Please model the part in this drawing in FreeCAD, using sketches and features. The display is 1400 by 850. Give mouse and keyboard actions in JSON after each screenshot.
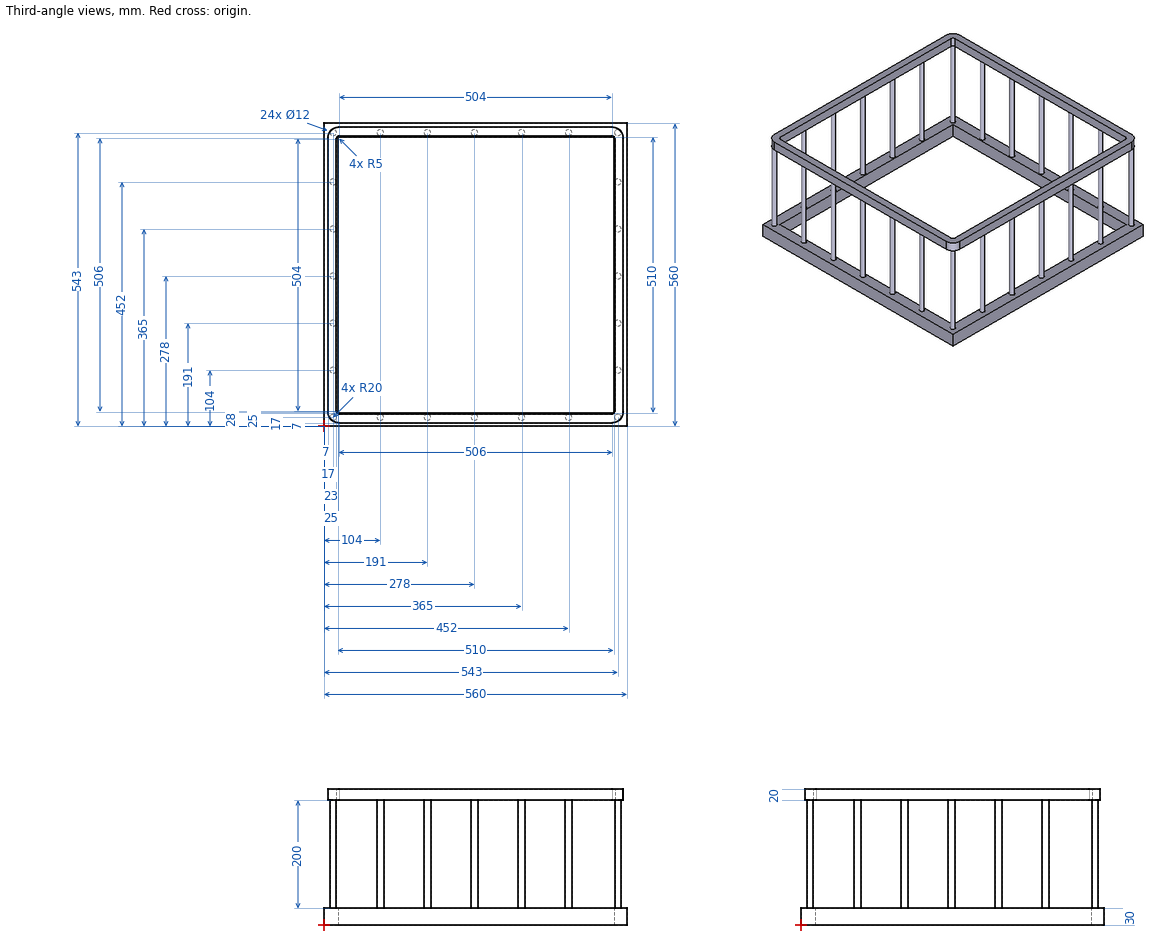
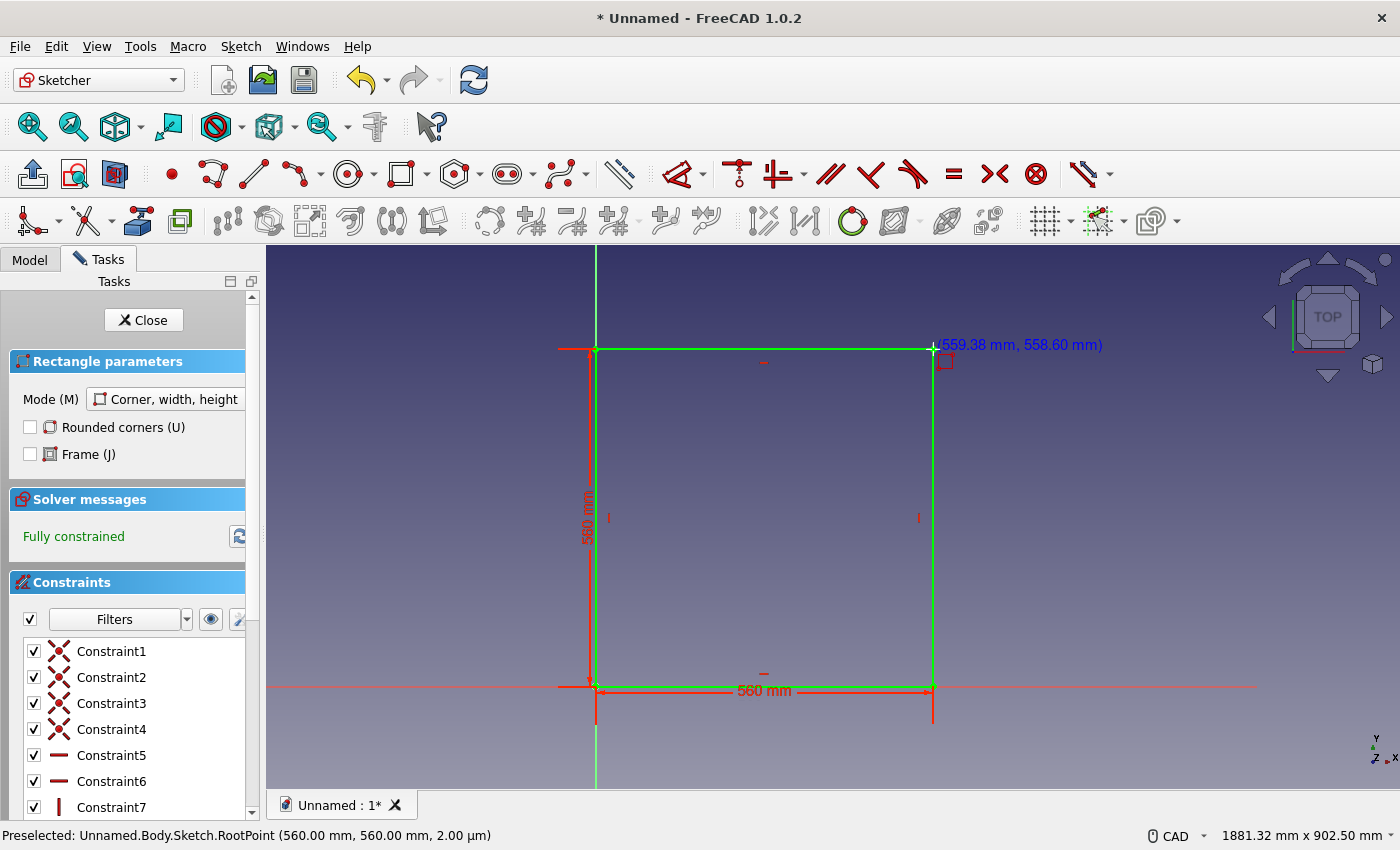
{"action": "left_click", "coordinate": [611, 364]}
{"action": "mouse_move", "coordinate": [918, 672]}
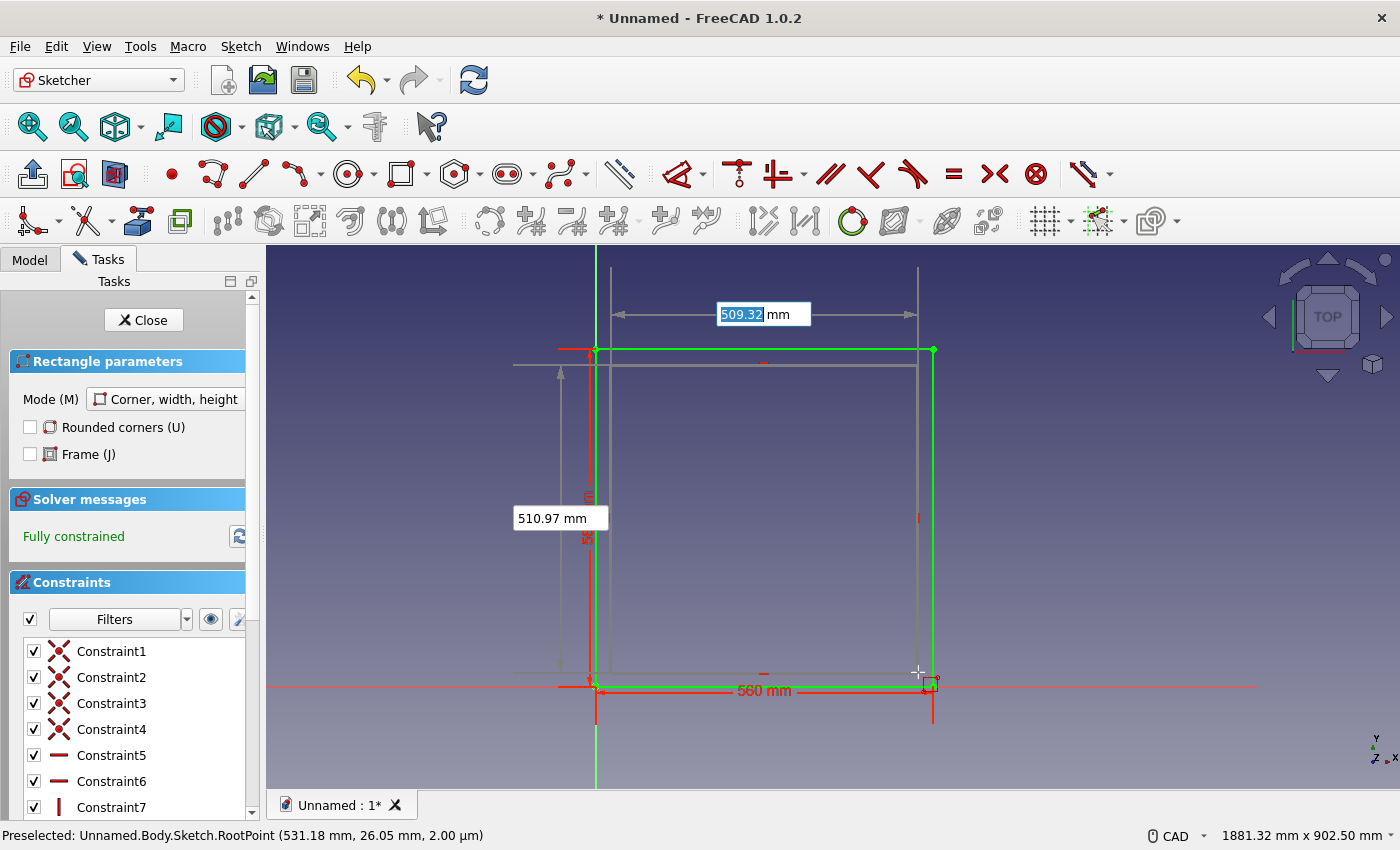
{"action": "type", "text": "510"}
{"action": "key", "text": "Tab"}
{"action": "type", "text": "510"}
{"action": "key", "text": "Return"}
{"action": "key", "text": "Escape"}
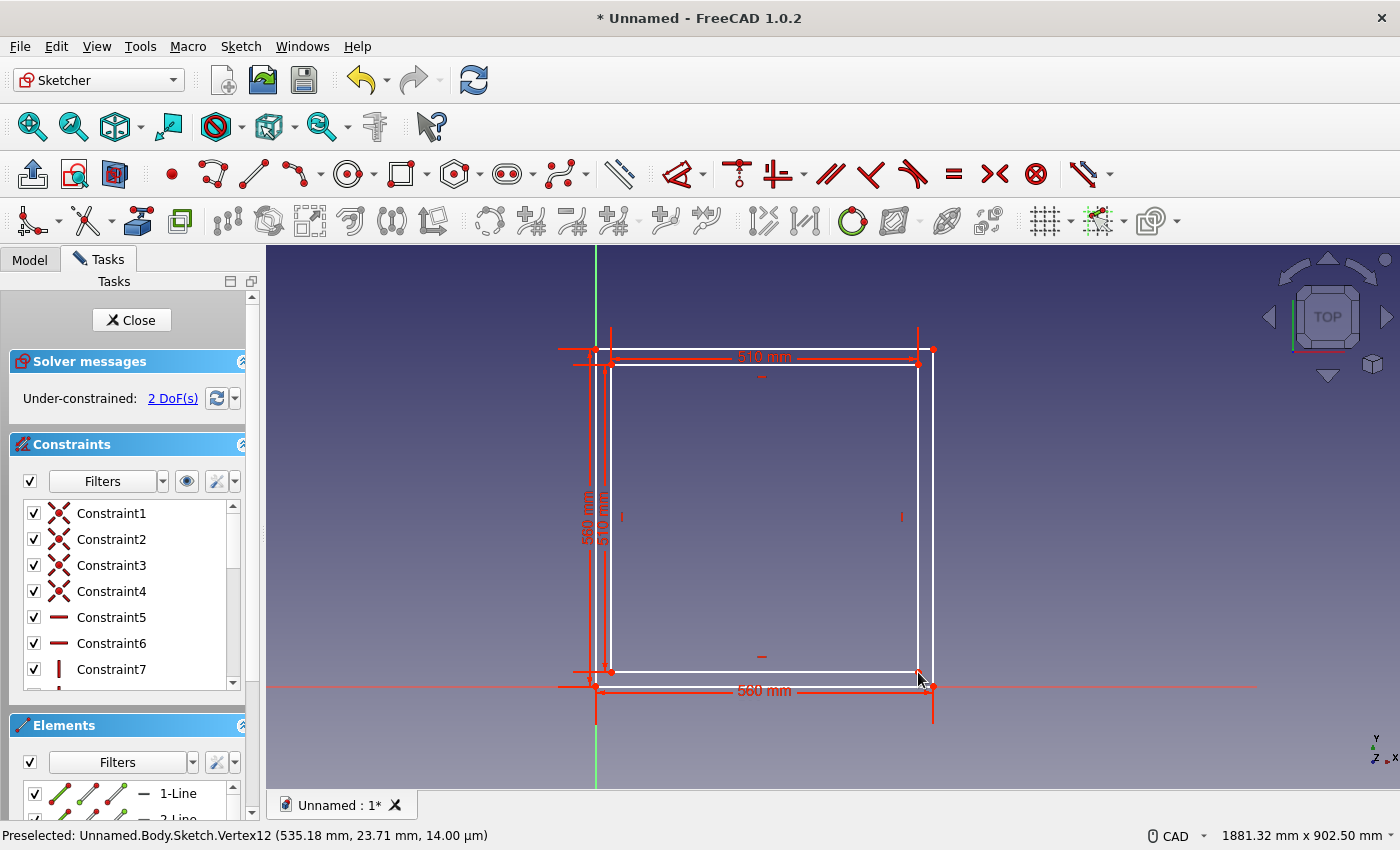
{"action": "left_click", "coordinate": [676, 174]}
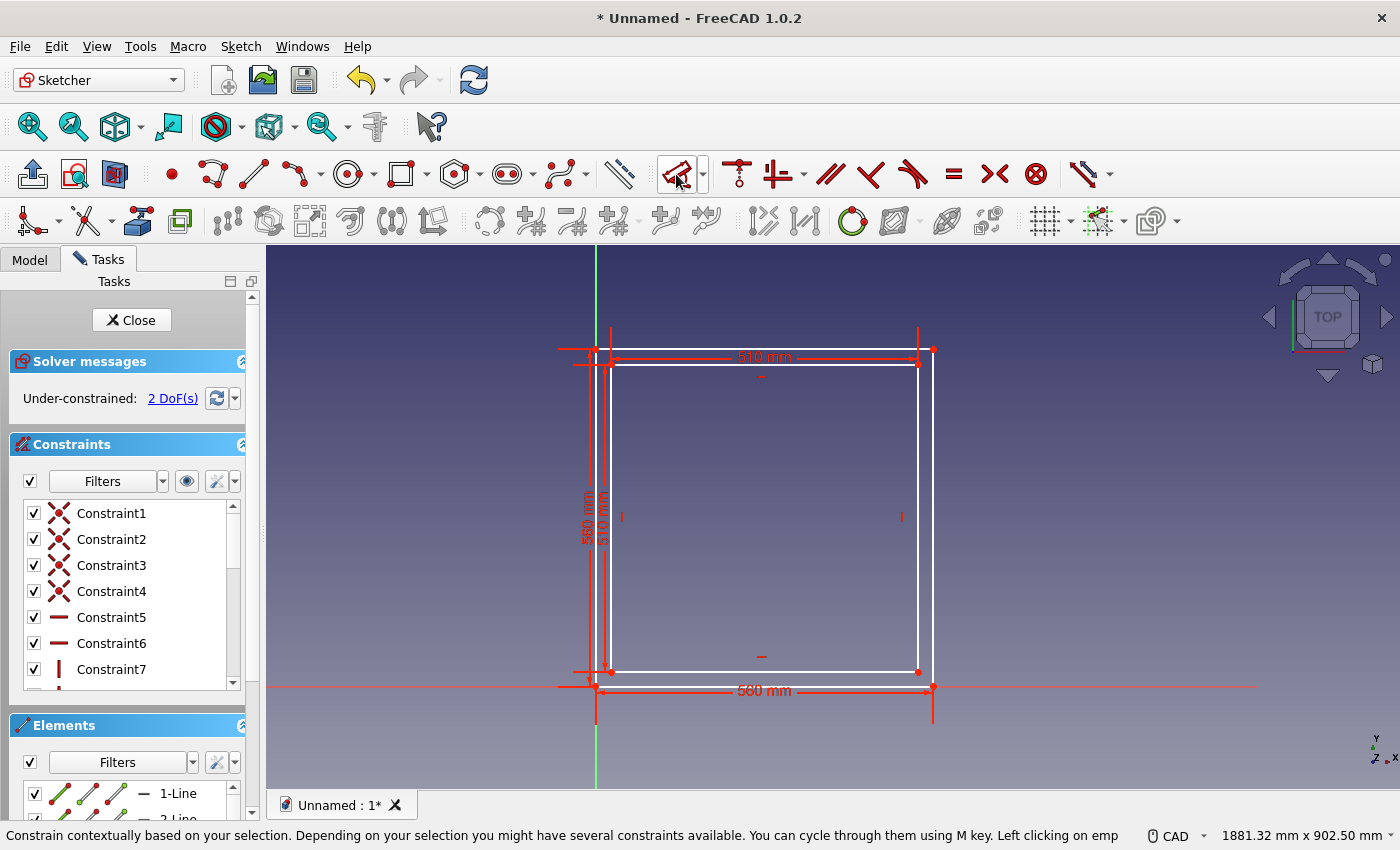
{"action": "scroll", "coordinate": [611, 365], "scroll_direction": "up", "scroll_amount": 5}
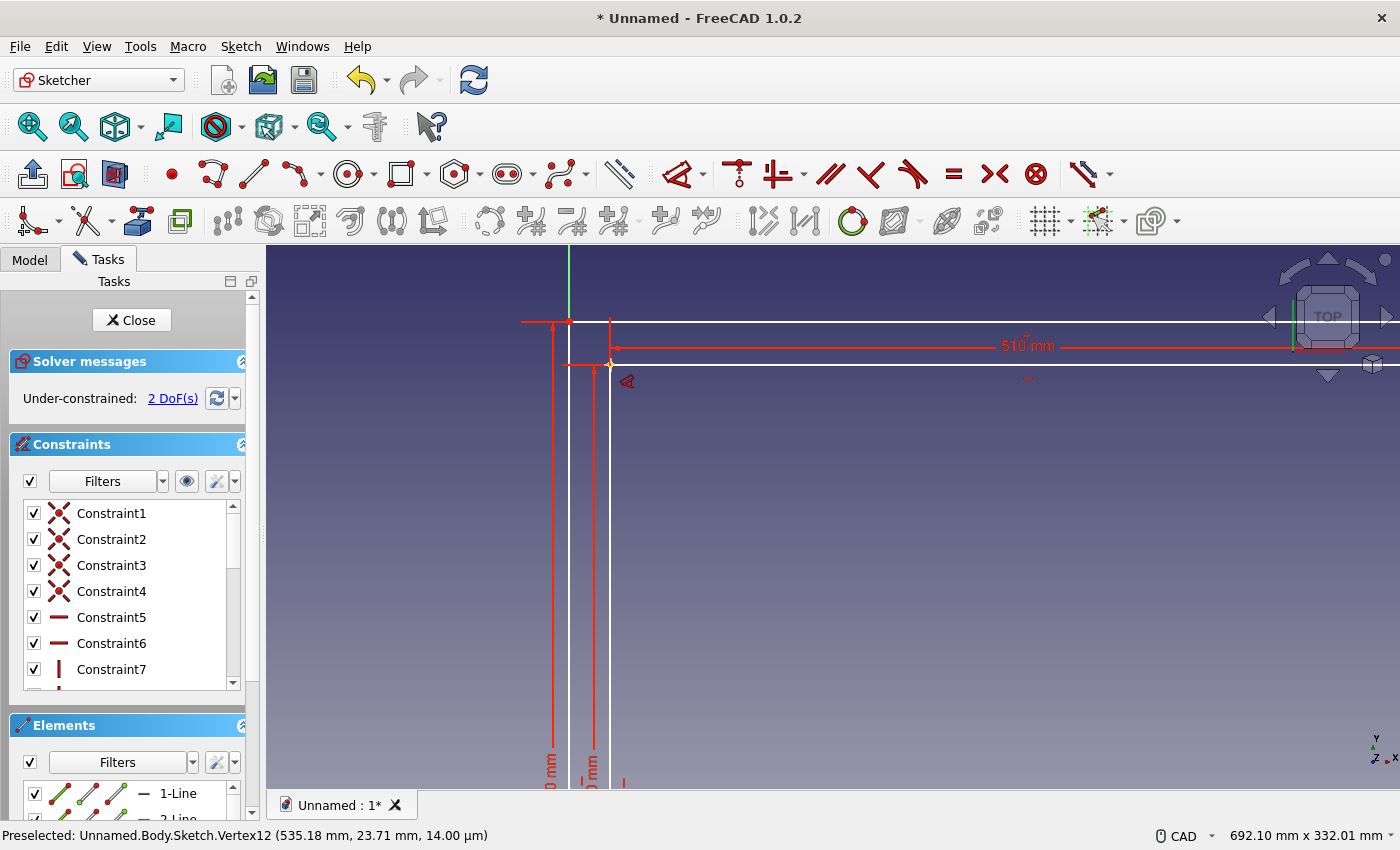
{"action": "left_click", "coordinate": [610, 365]}
{"action": "left_click", "coordinate": [590, 307]}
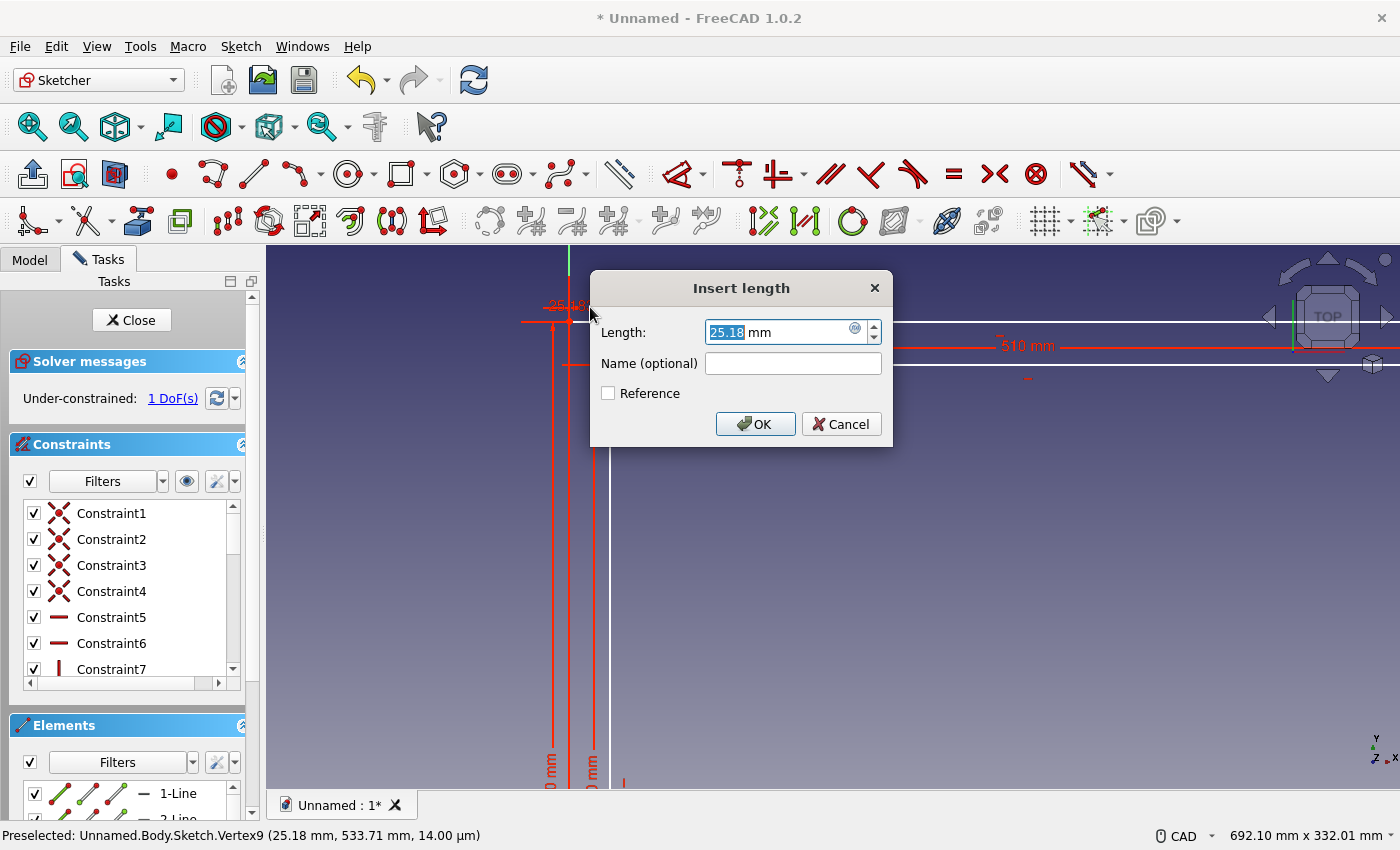
{"action": "type", "text": "25"}
{"action": "key", "text": "Return"}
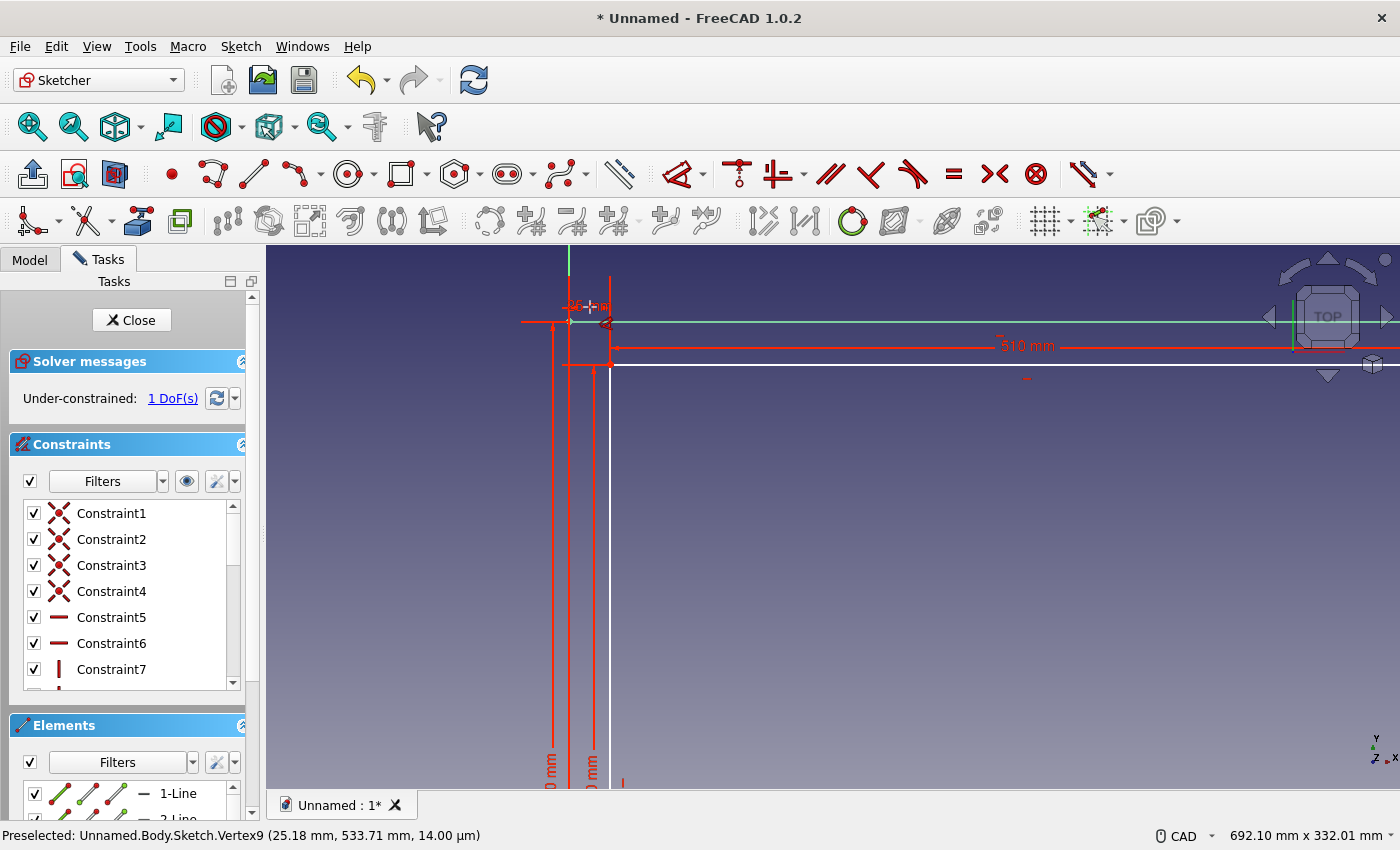
{"action": "scroll", "coordinate": [611, 364], "scroll_direction": "down", "scroll_amount": 5}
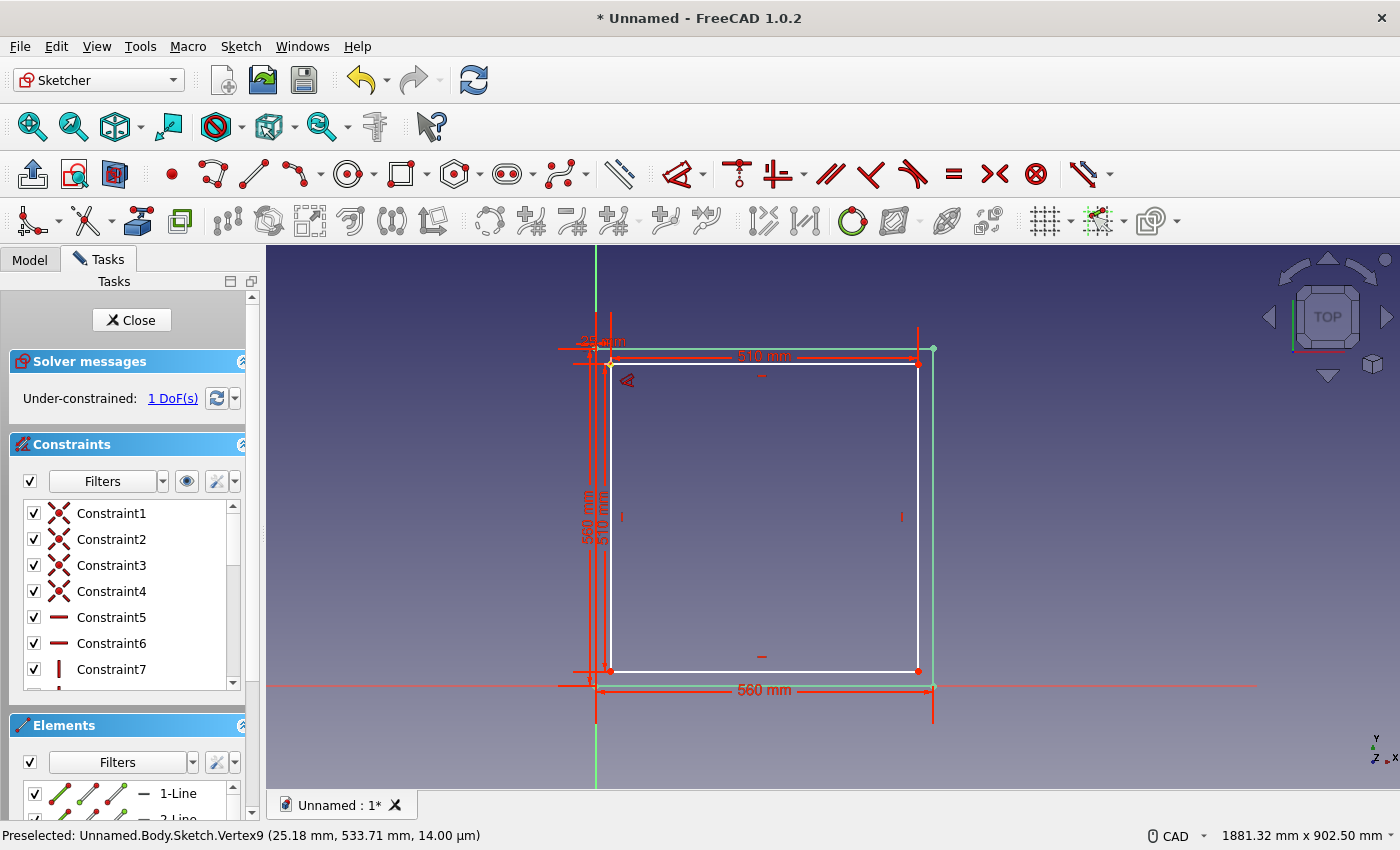
{"action": "scroll", "coordinate": [611, 672], "scroll_direction": "up", "scroll_amount": 5}